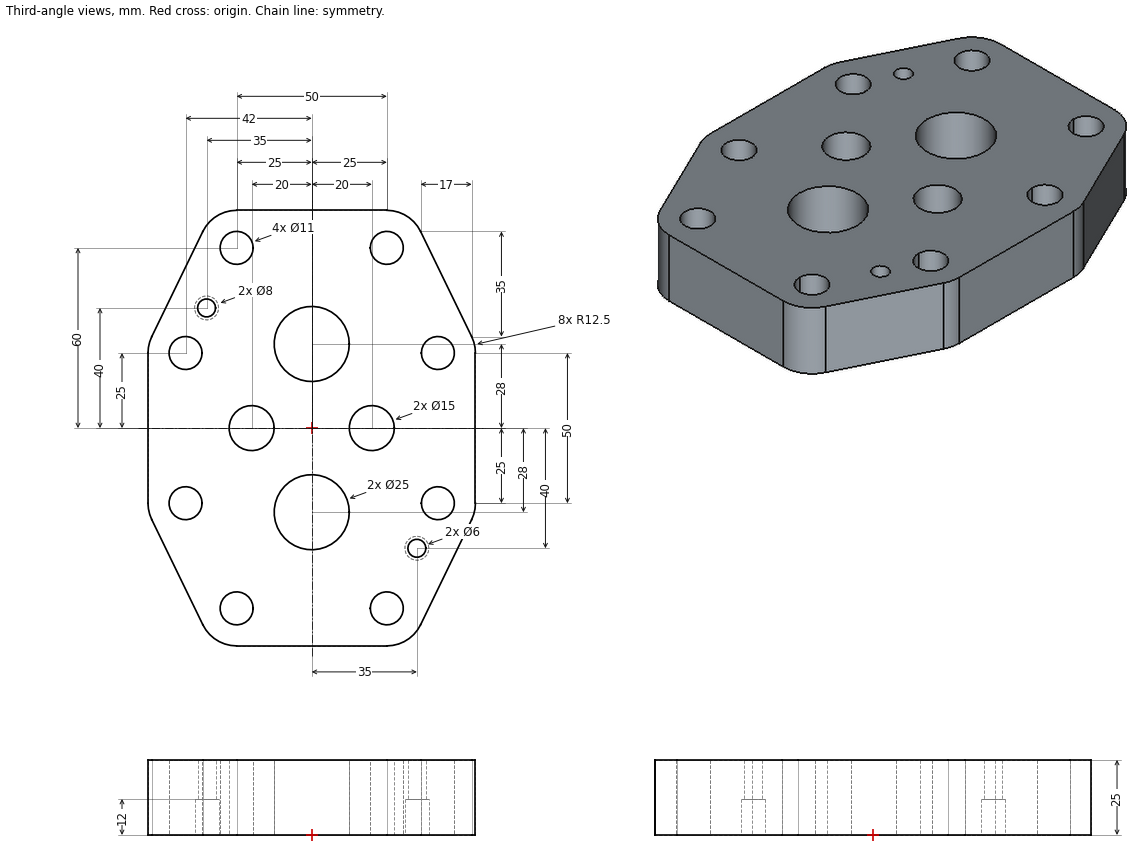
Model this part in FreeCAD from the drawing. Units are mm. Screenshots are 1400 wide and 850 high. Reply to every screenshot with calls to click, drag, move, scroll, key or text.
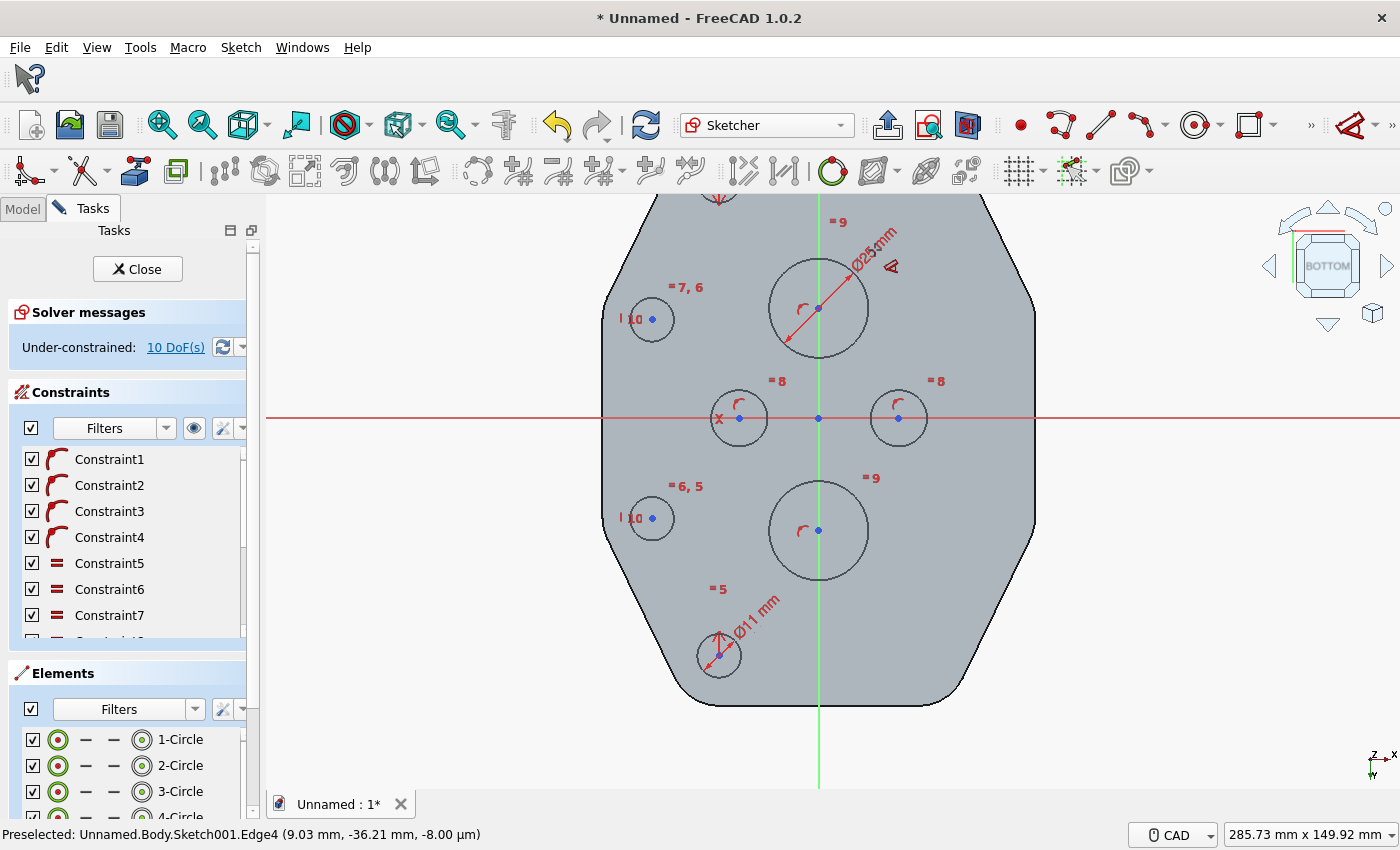
click(919, 398)
click(942, 375)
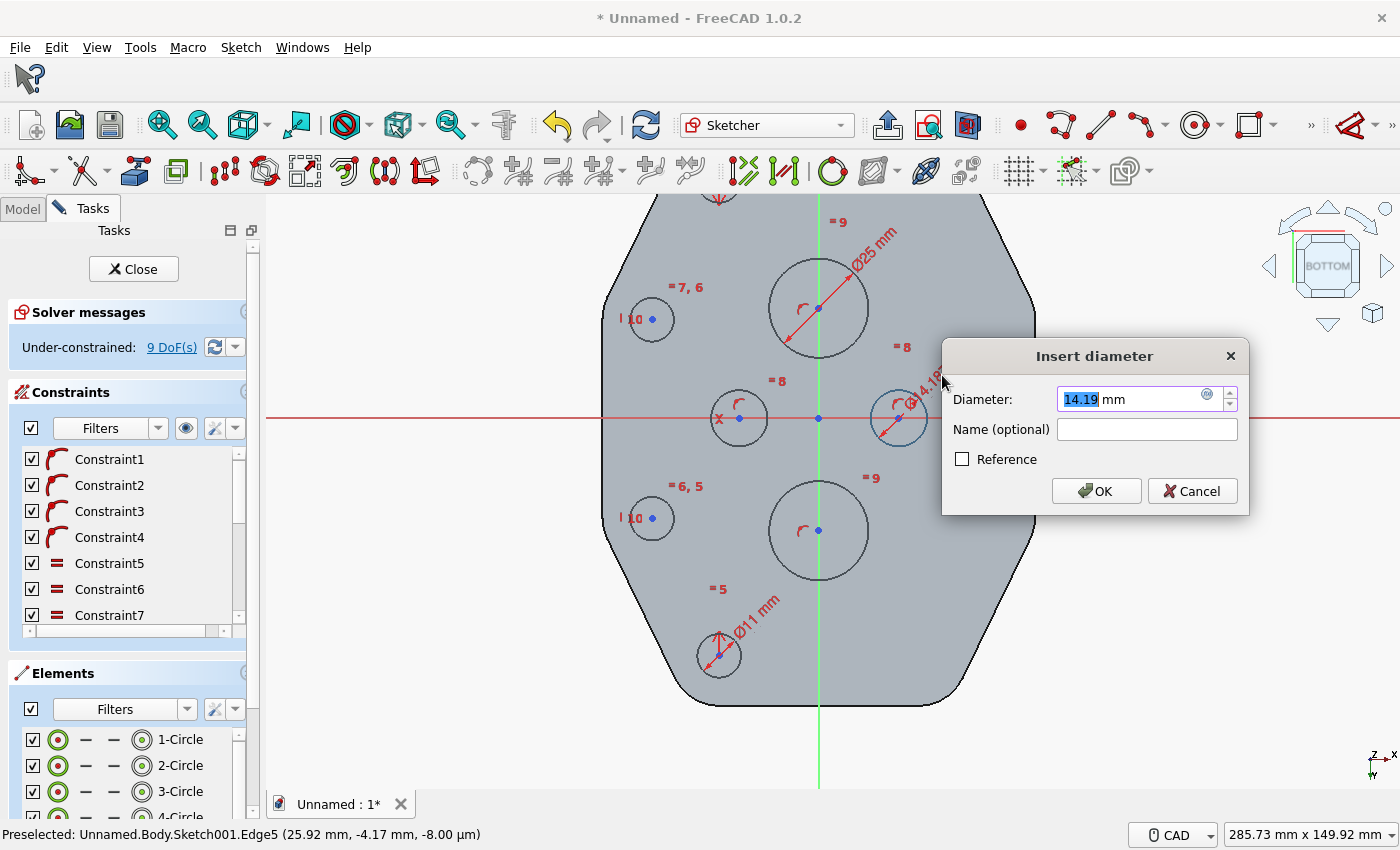
text(15)
key(Return)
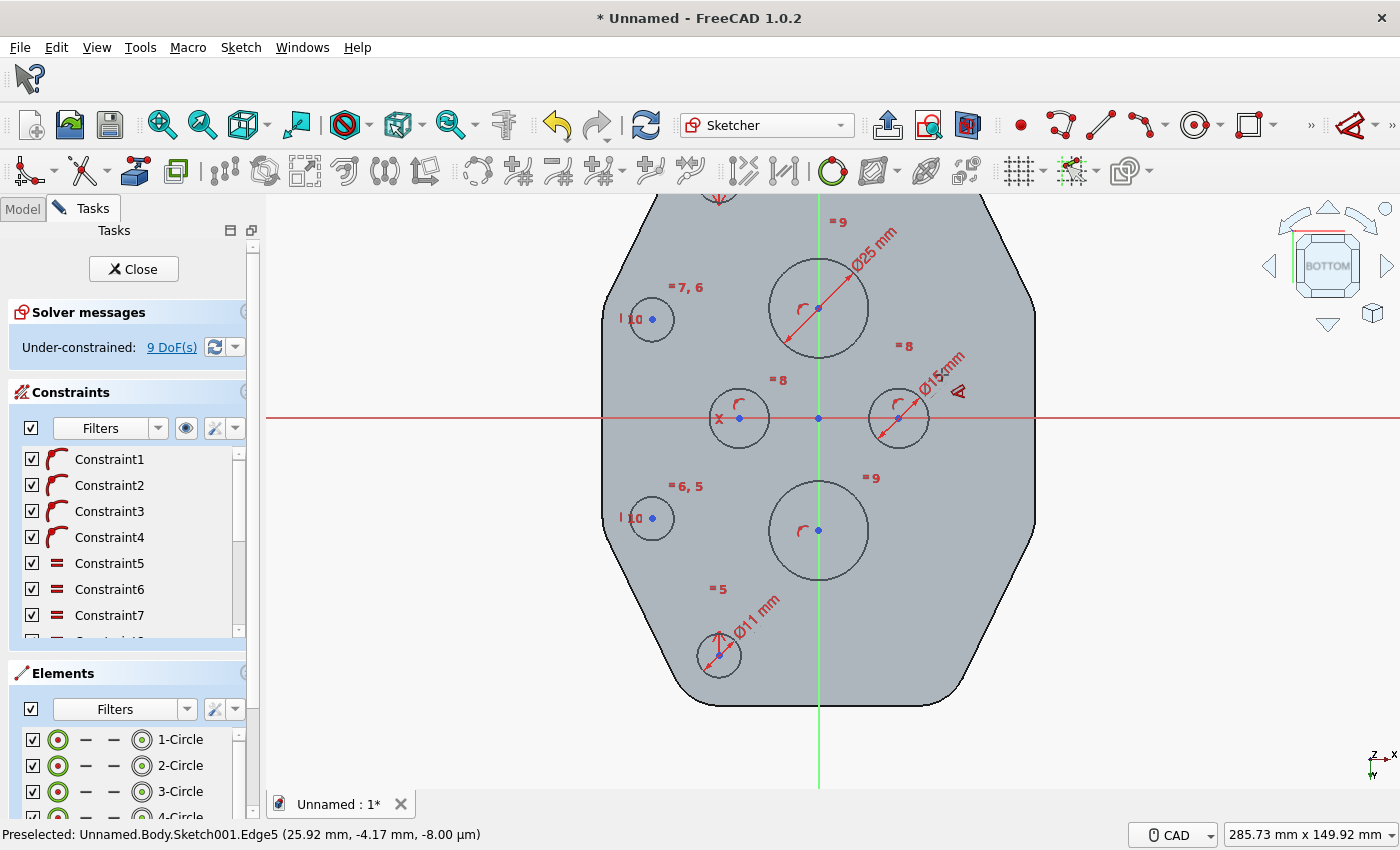
click(719, 656)
click(769, 690)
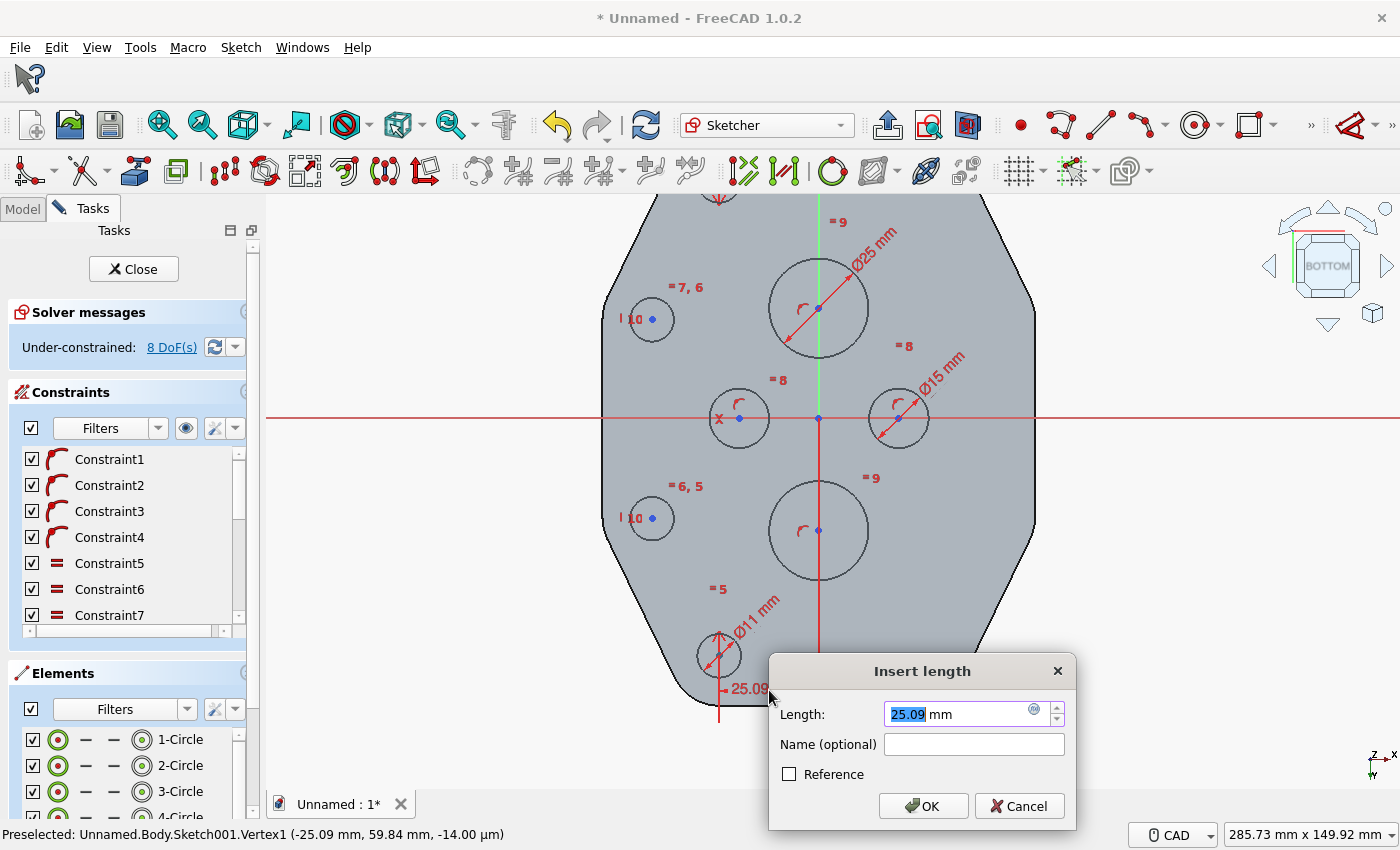
text(25)
key(Return)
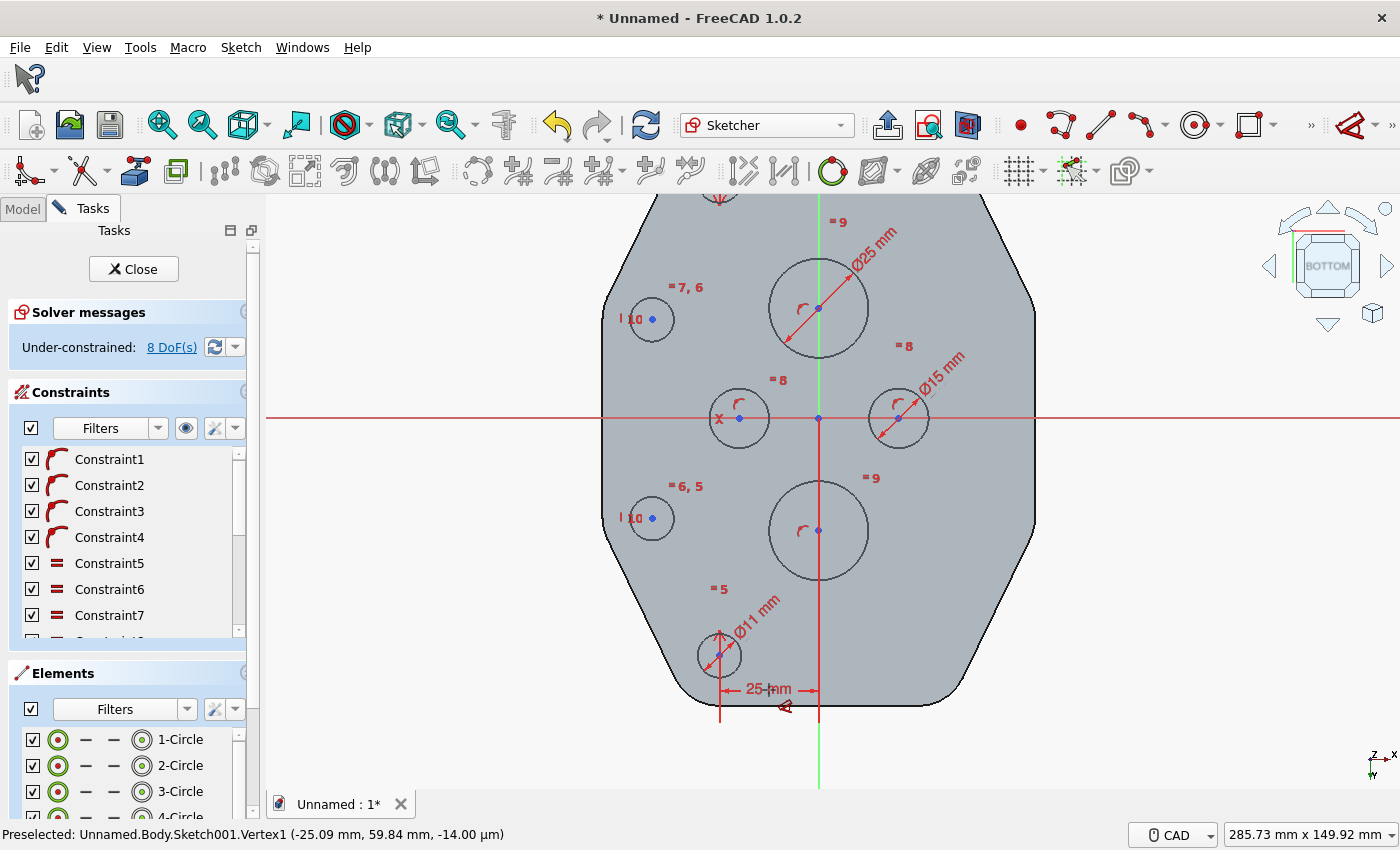
click(720, 656)
click(686, 537)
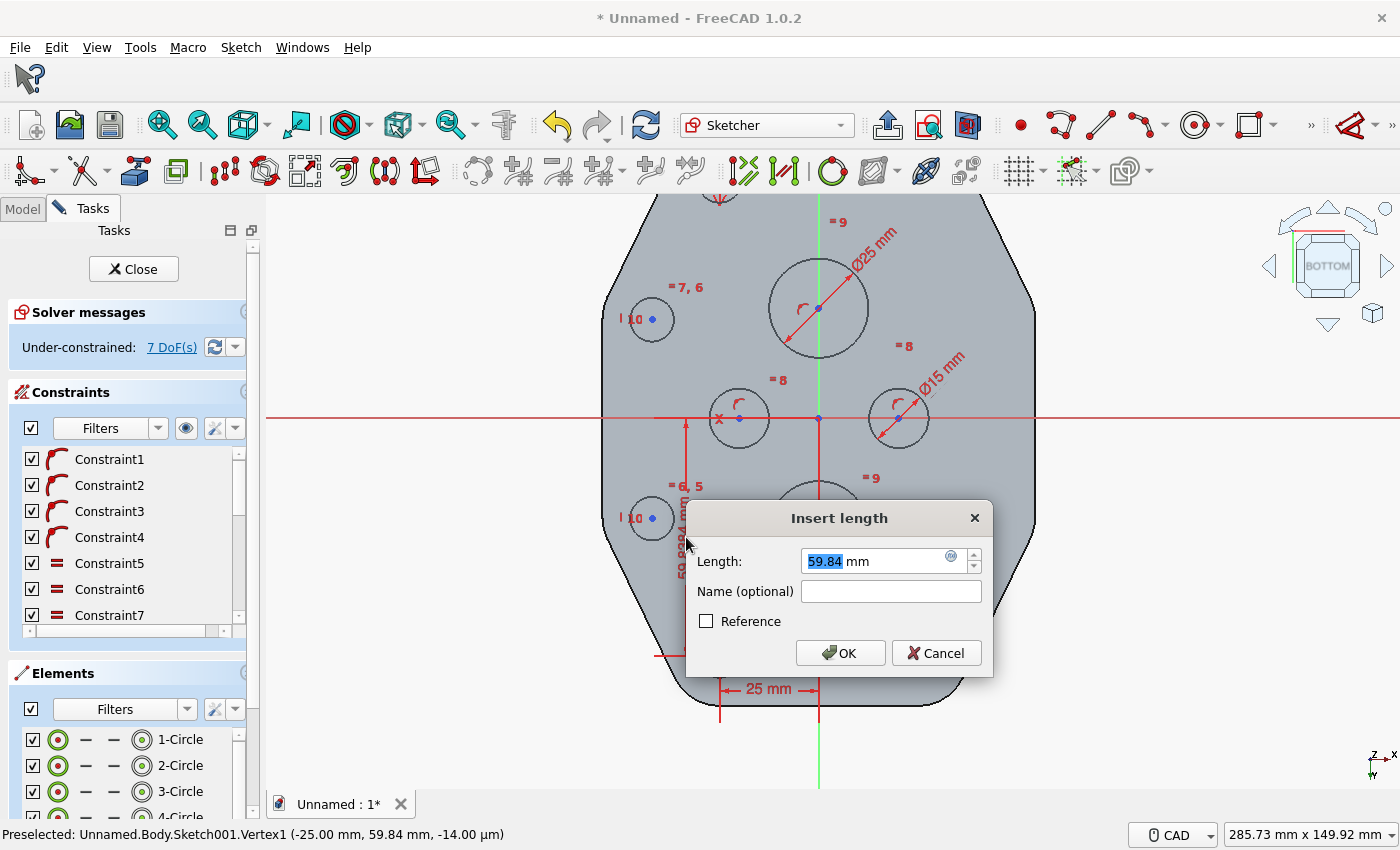
text(60)
key(Return)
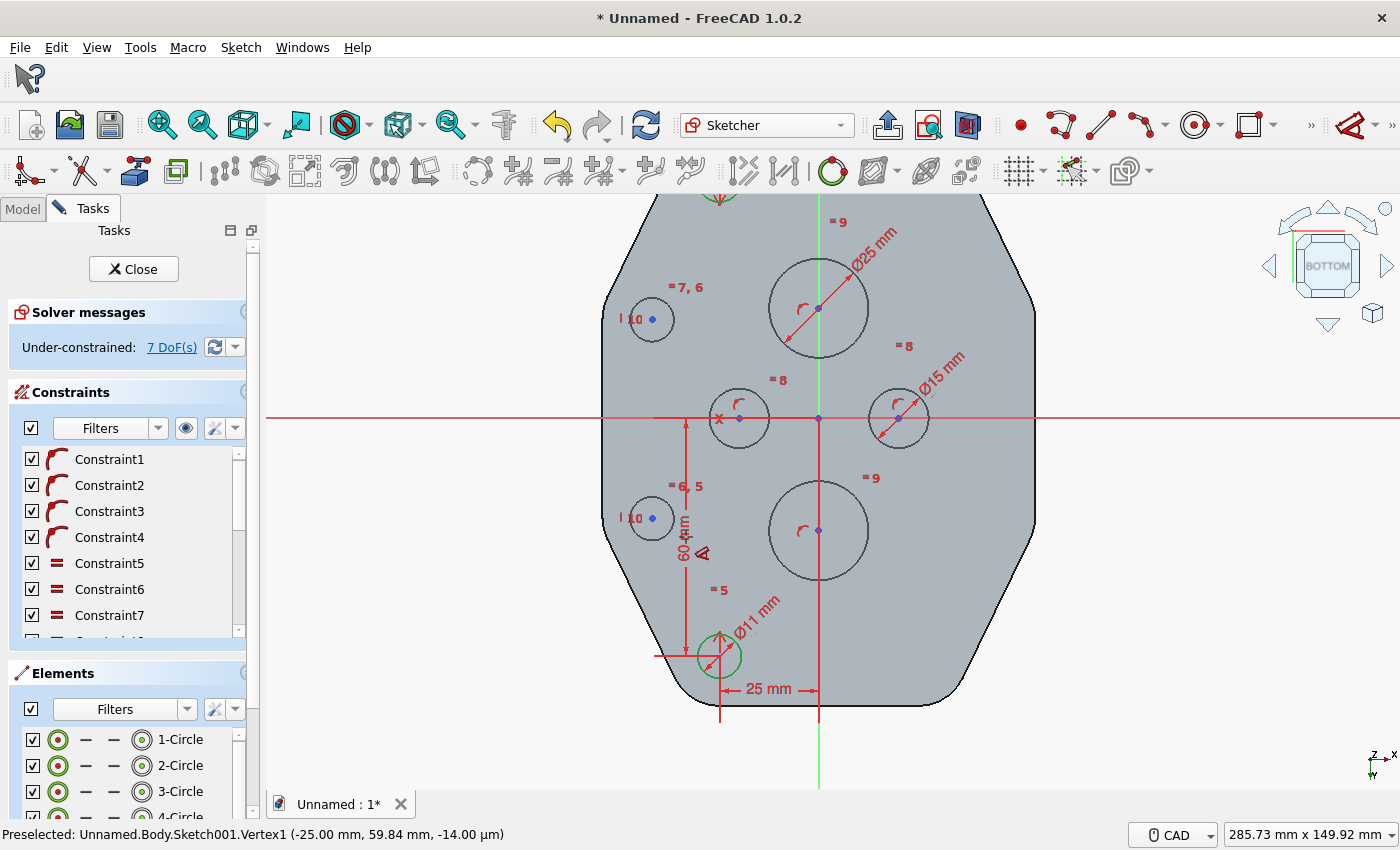
click(652, 519)
click(794, 553)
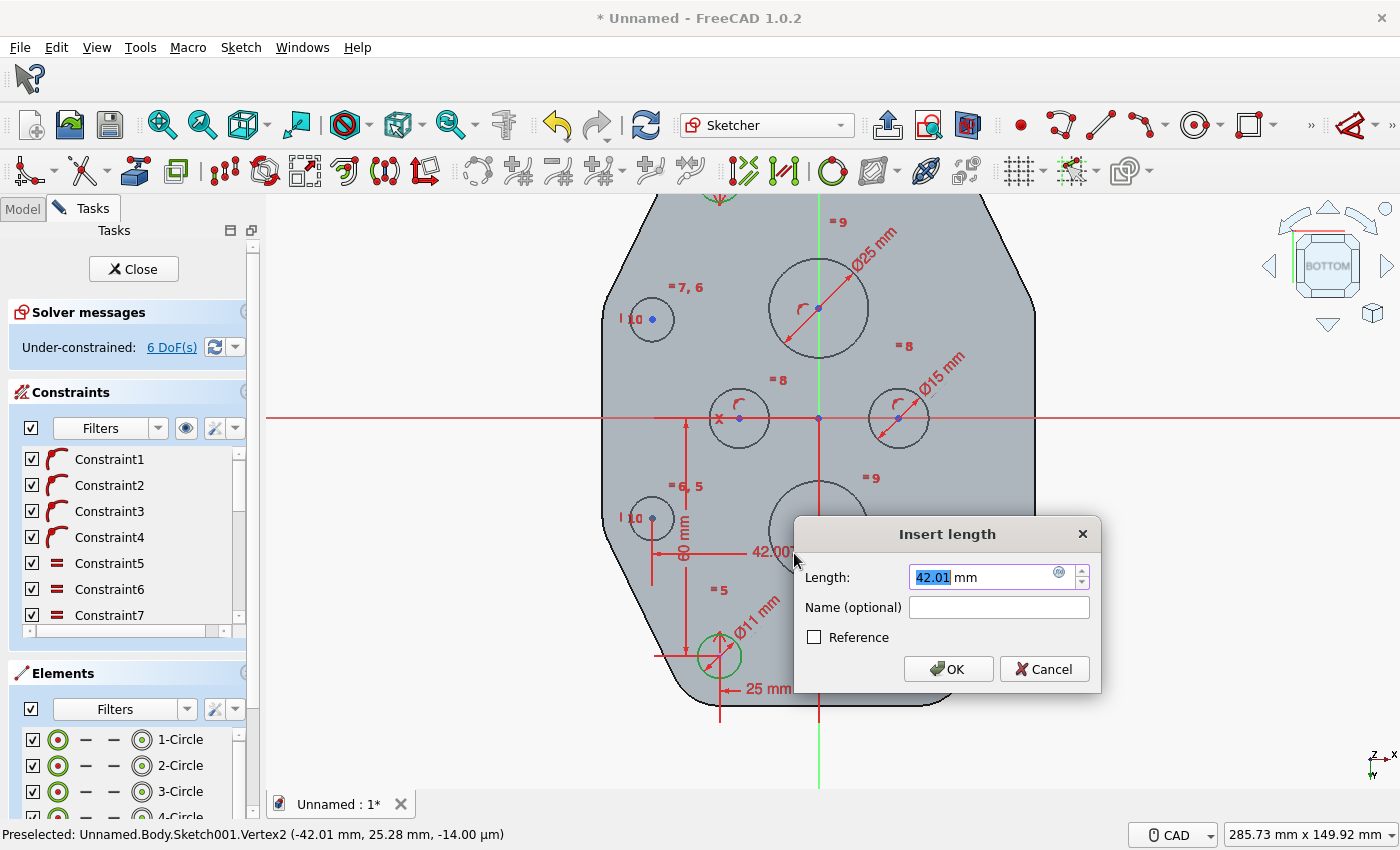
text(42)
key(Return)